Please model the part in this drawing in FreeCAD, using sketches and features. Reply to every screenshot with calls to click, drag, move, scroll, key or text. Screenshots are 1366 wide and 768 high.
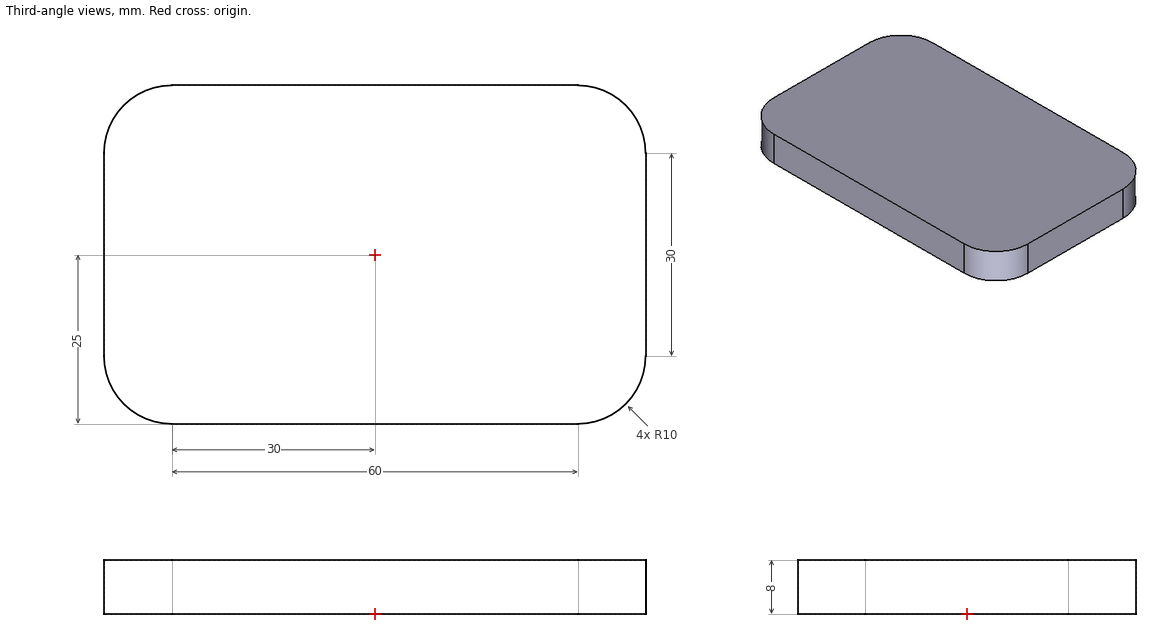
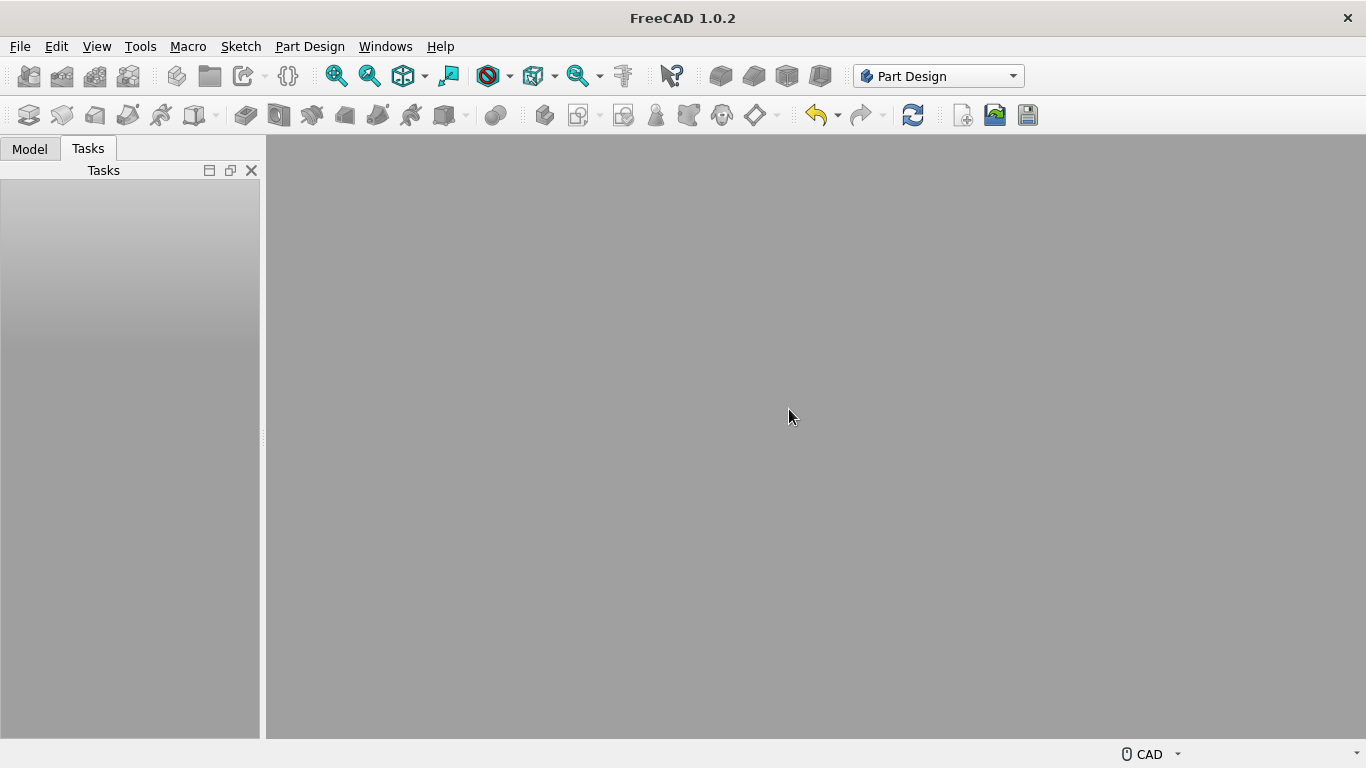
key(ctrl+n)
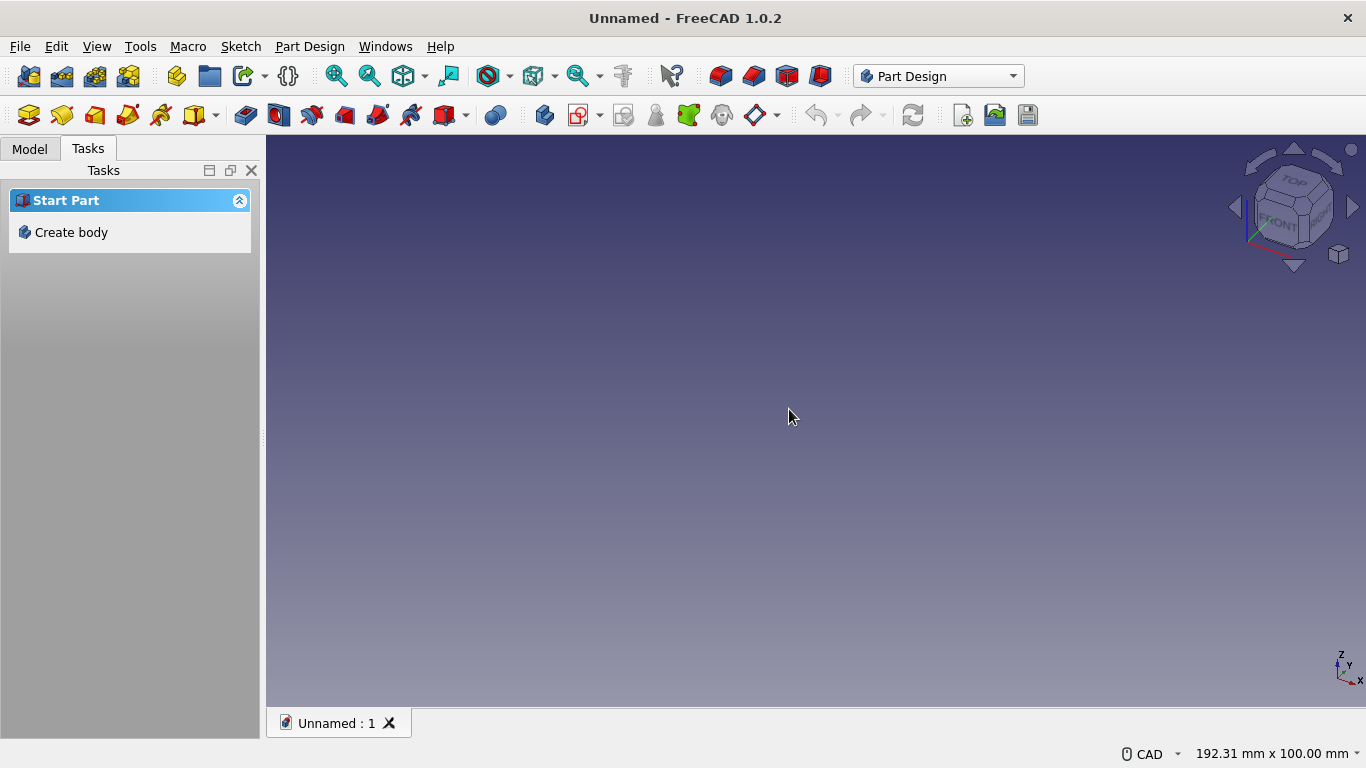
click(578, 116)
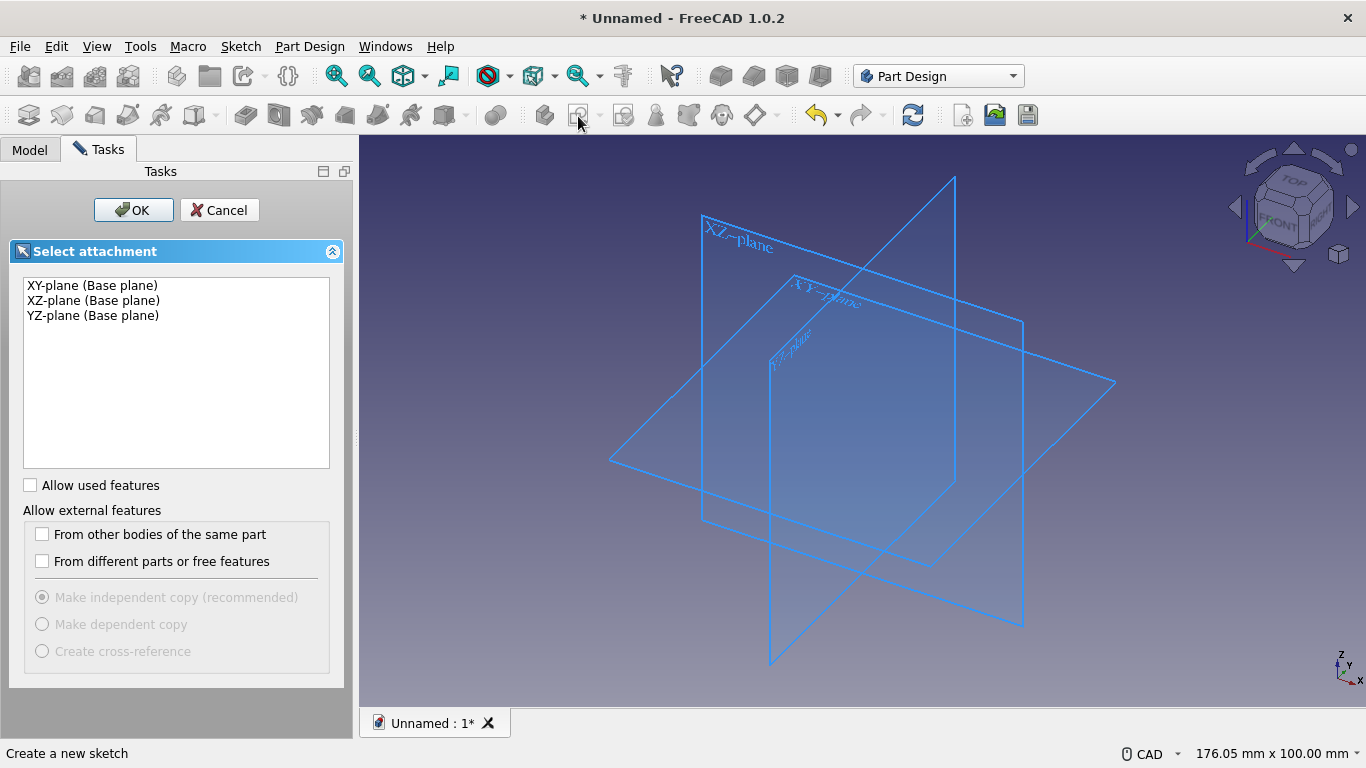
click(84, 286)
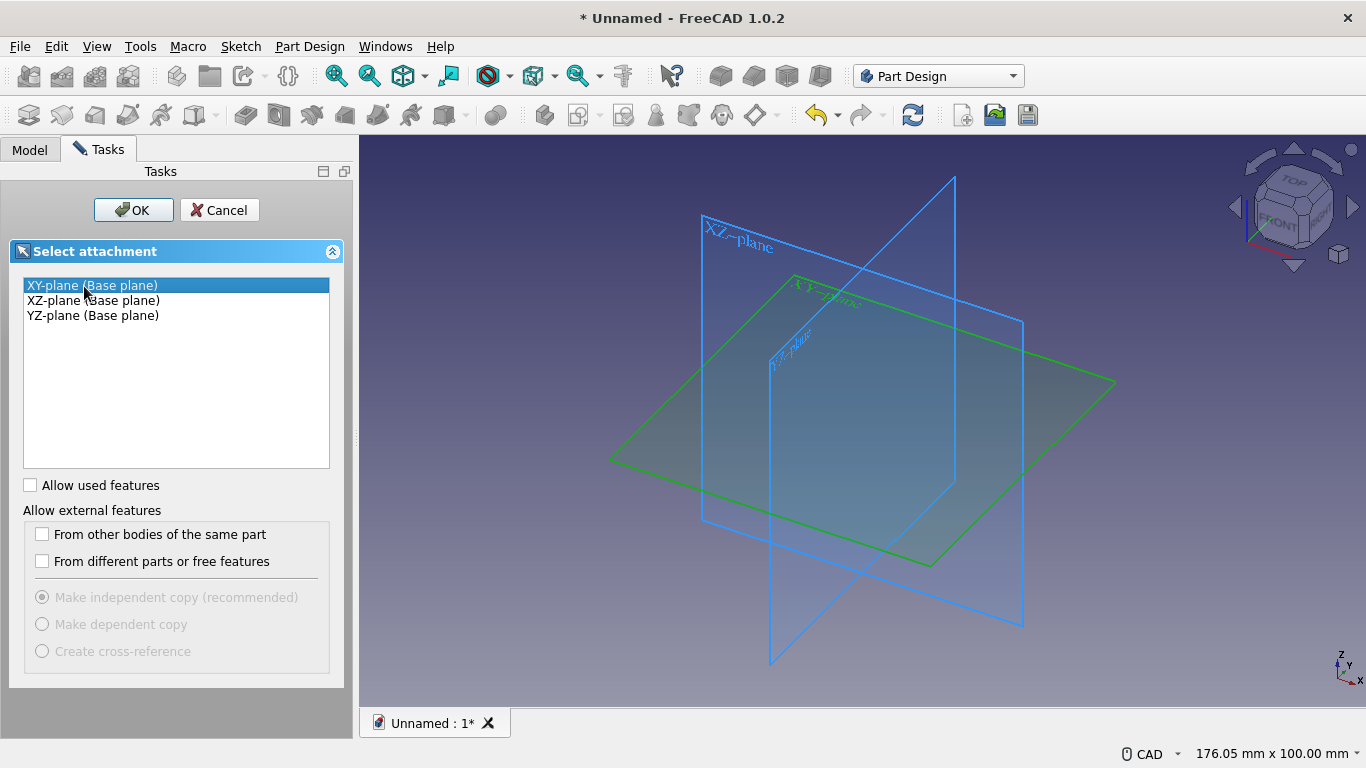
click(134, 210)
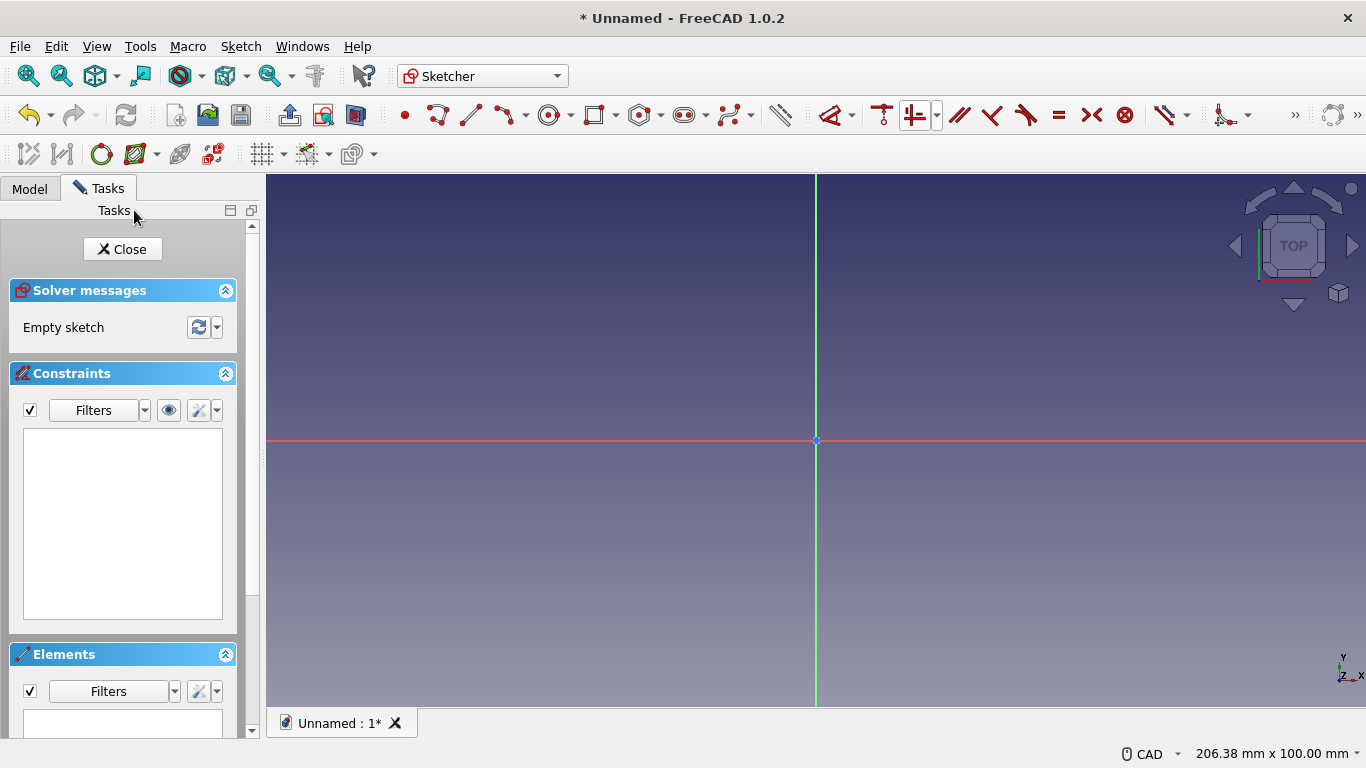
key(g)
key(l)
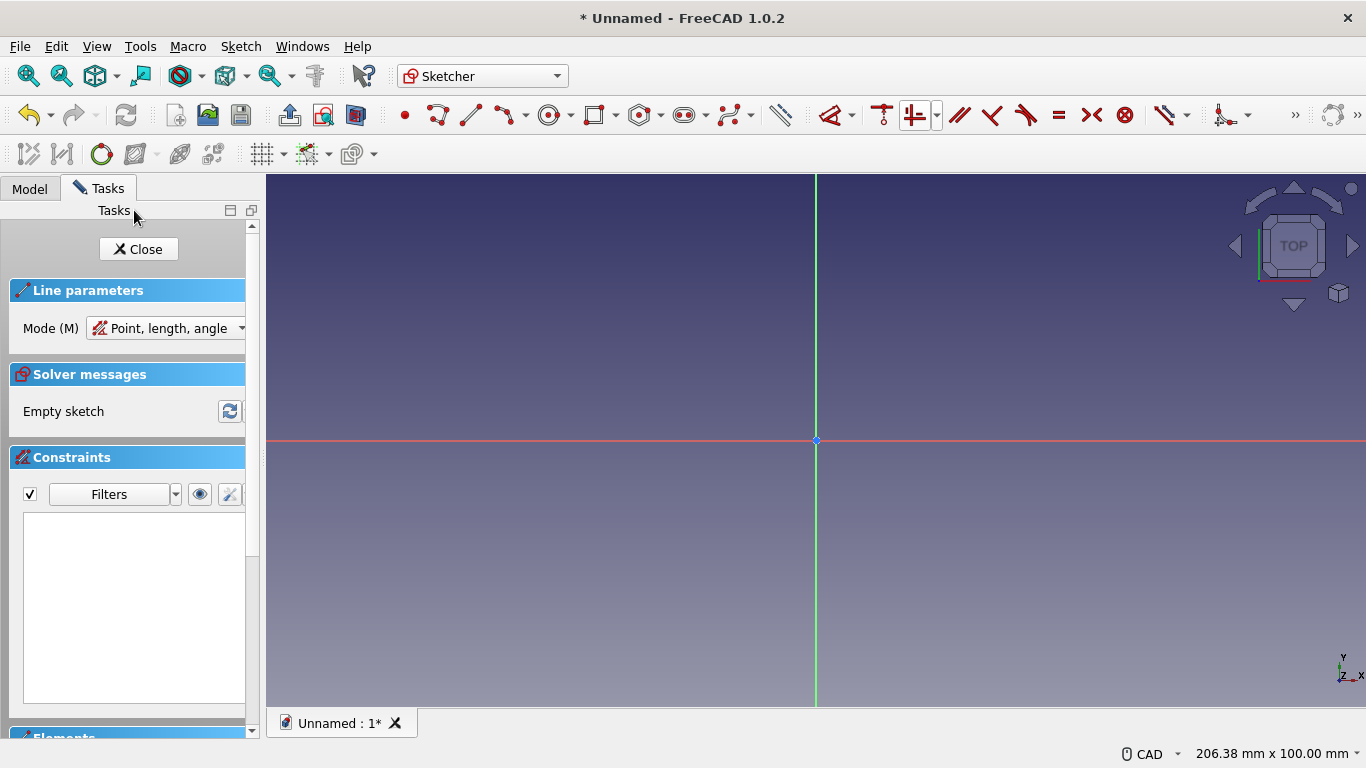
click(656, 574)
click(976, 574)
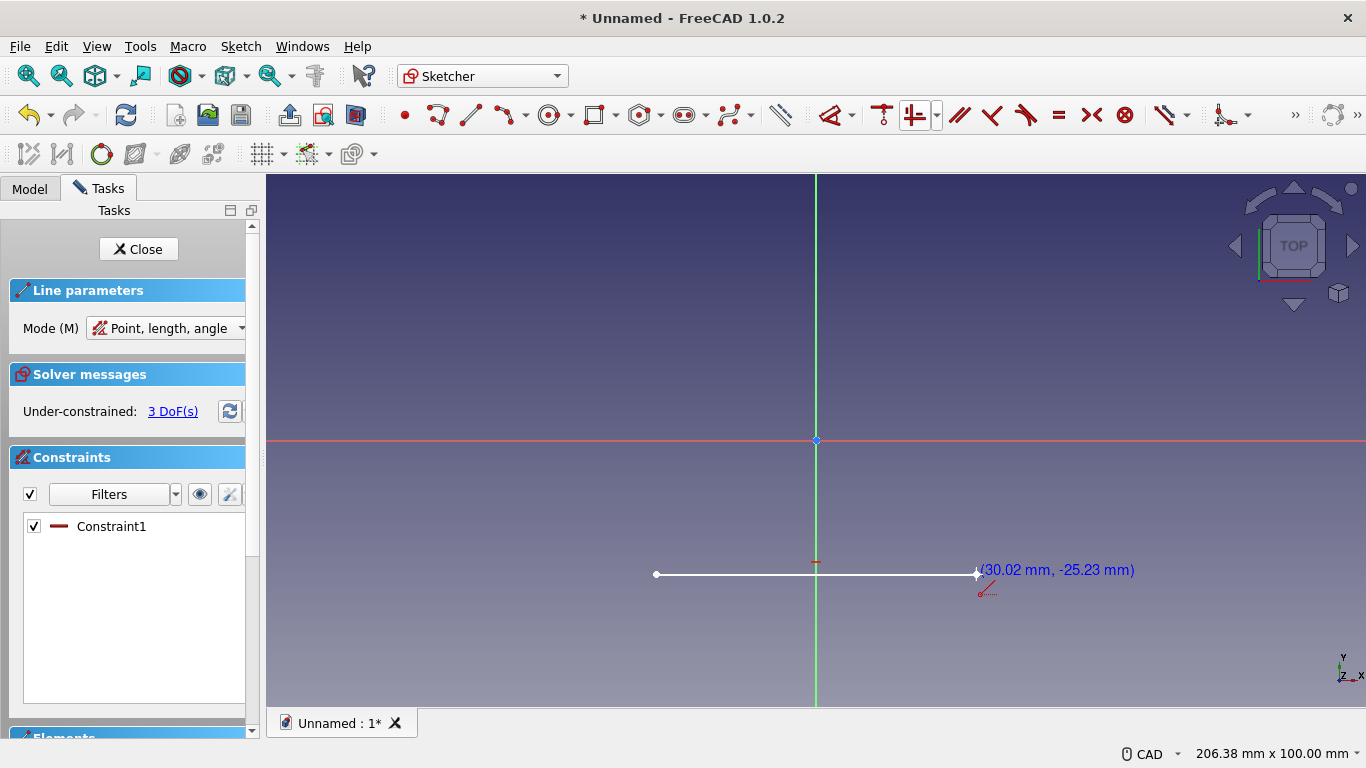
click(1029, 520)
click(1029, 361)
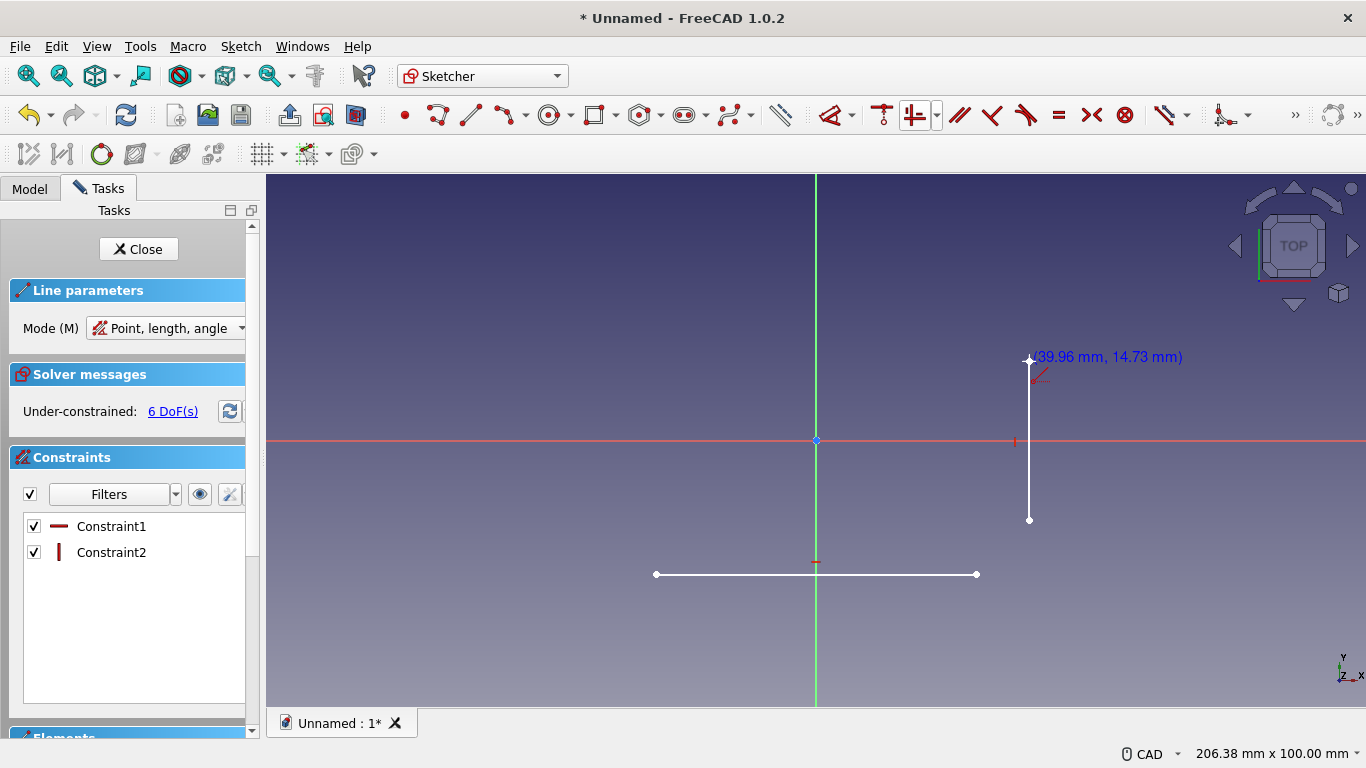
click(976, 307)
click(656, 307)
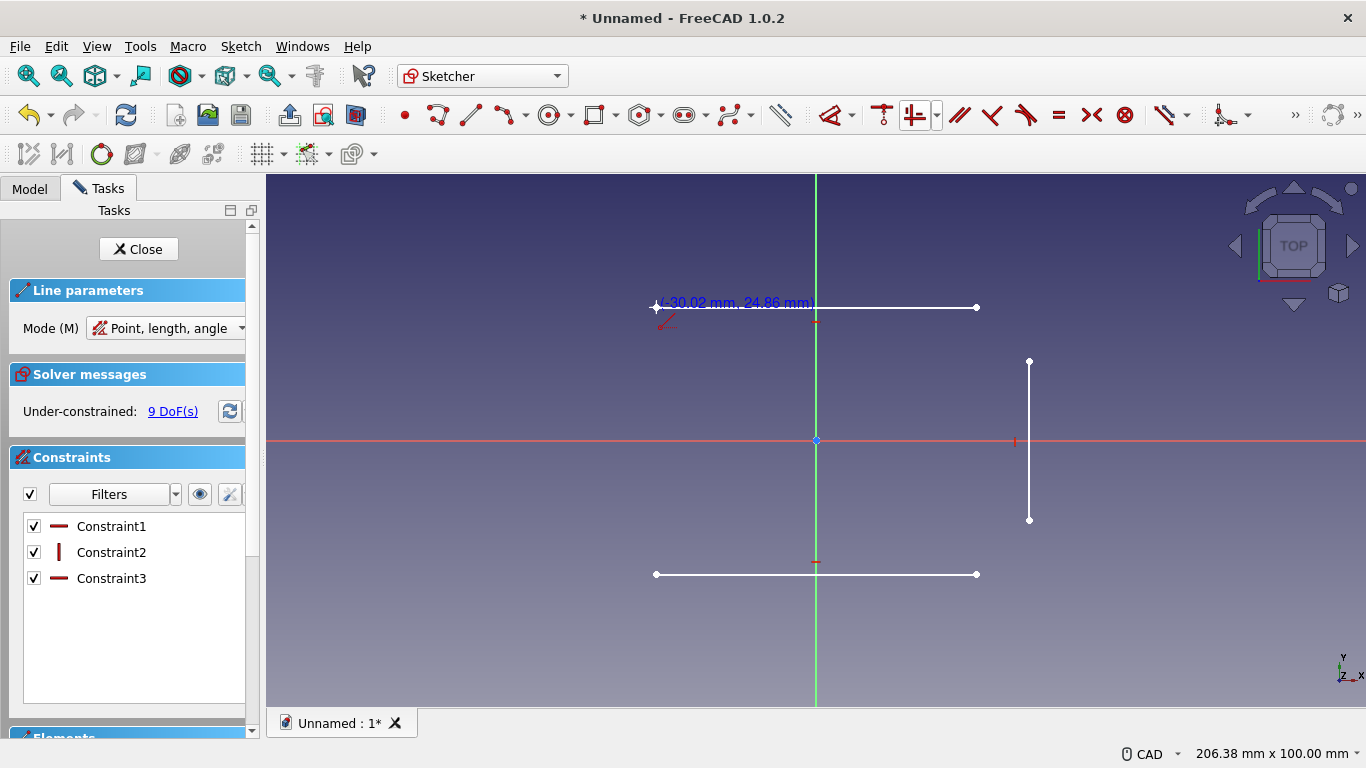
click(603, 361)
click(603, 520)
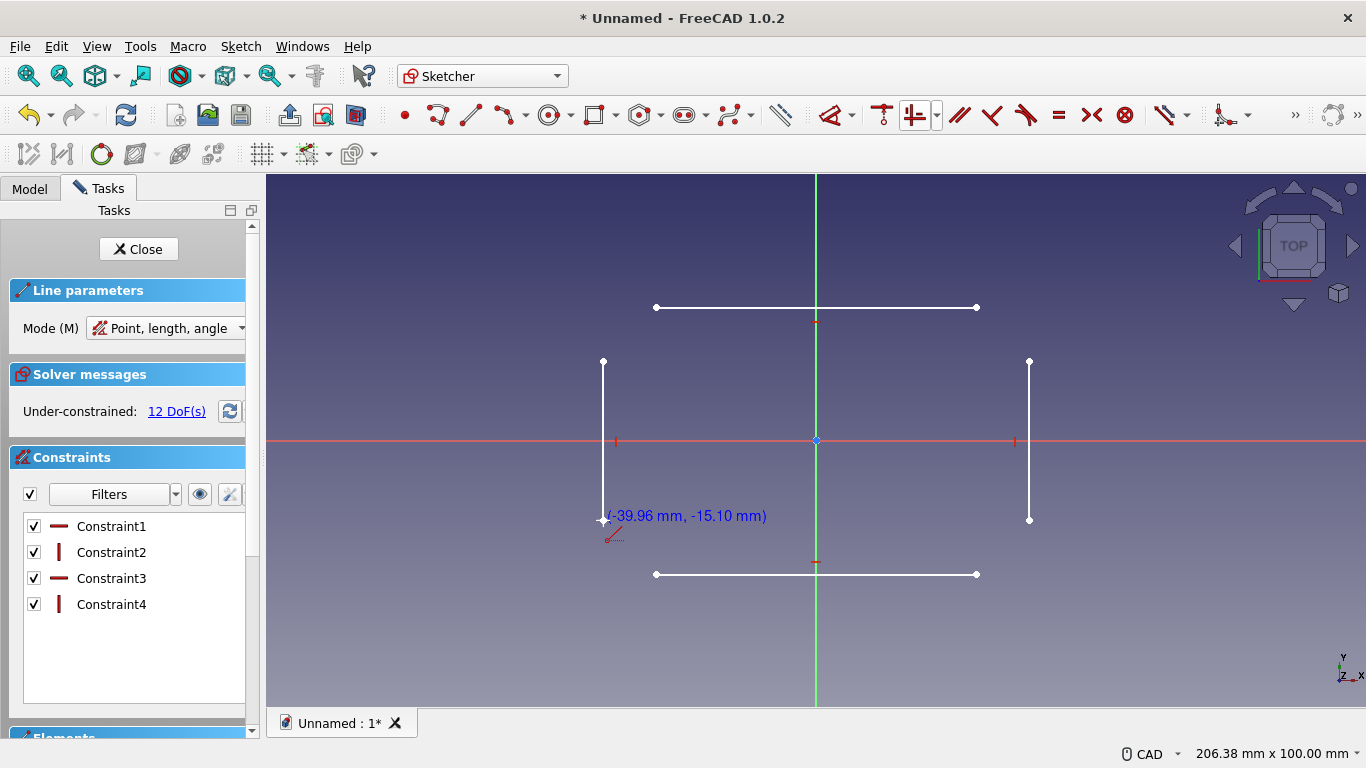
key(g)
key(3)
key(a)